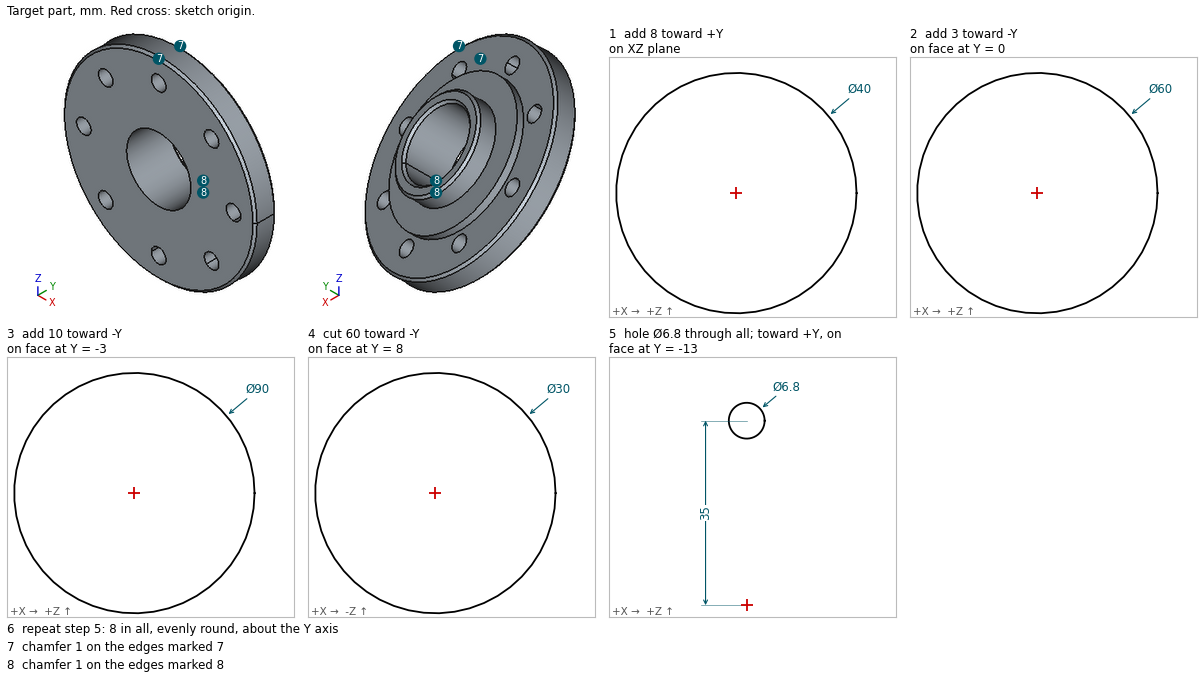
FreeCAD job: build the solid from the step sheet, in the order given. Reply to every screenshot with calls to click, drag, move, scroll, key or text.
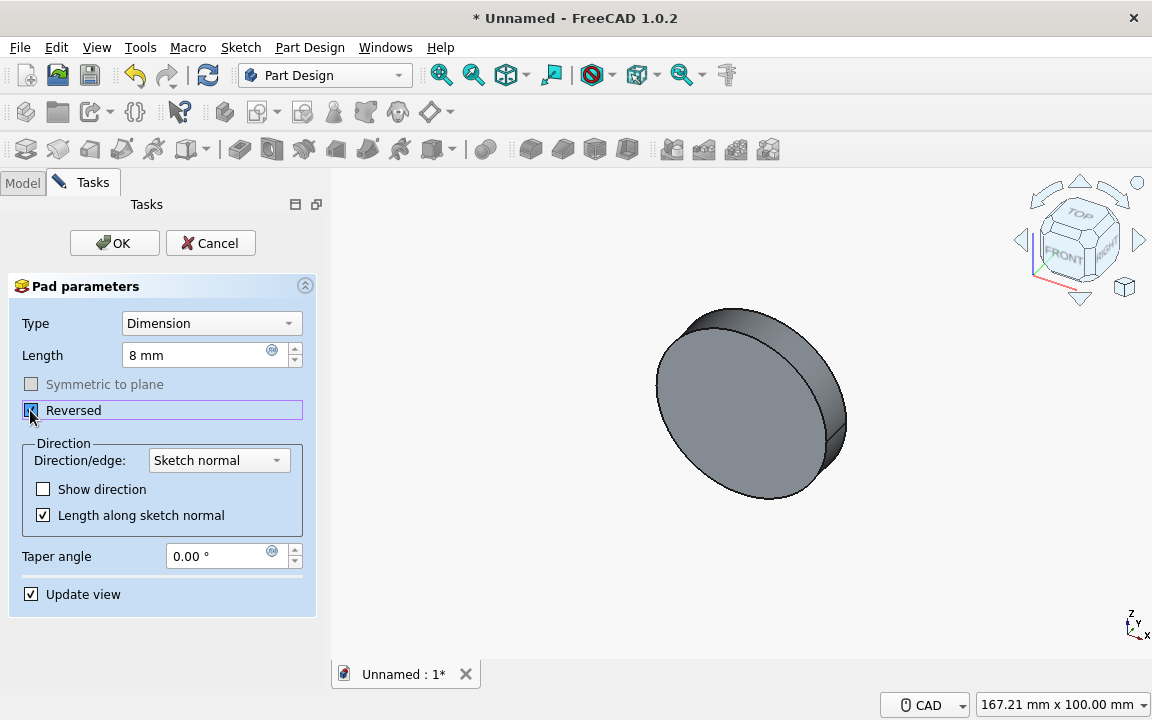
click(115, 243)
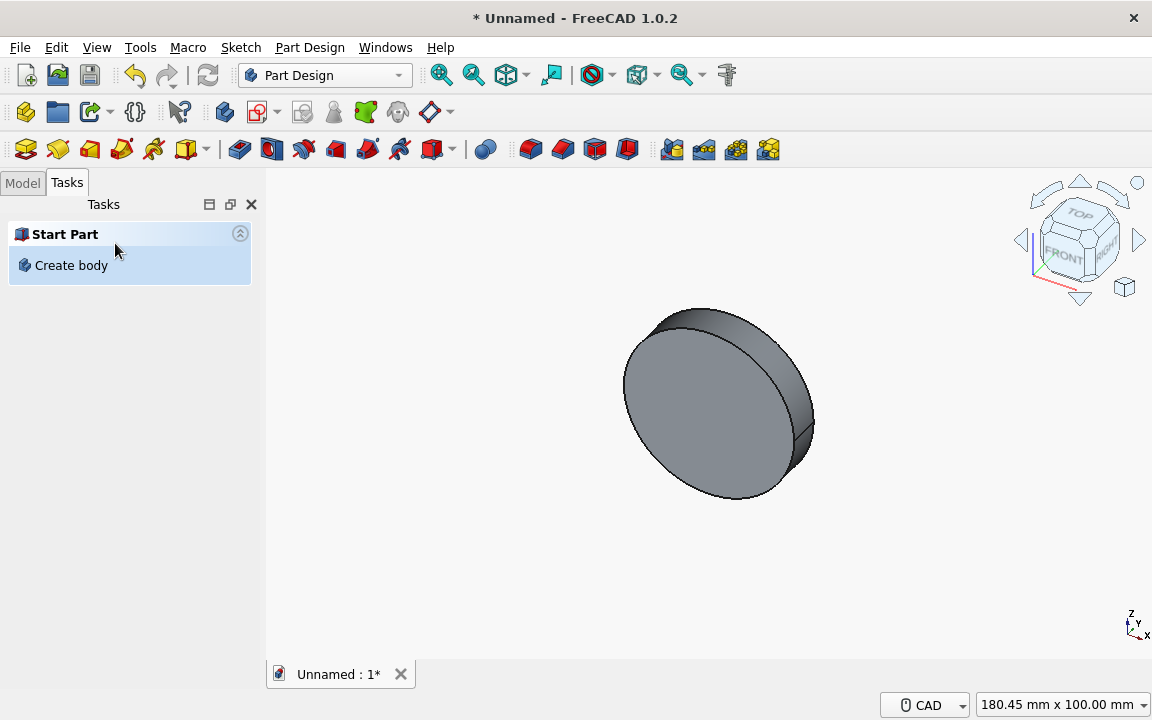
click(709, 412)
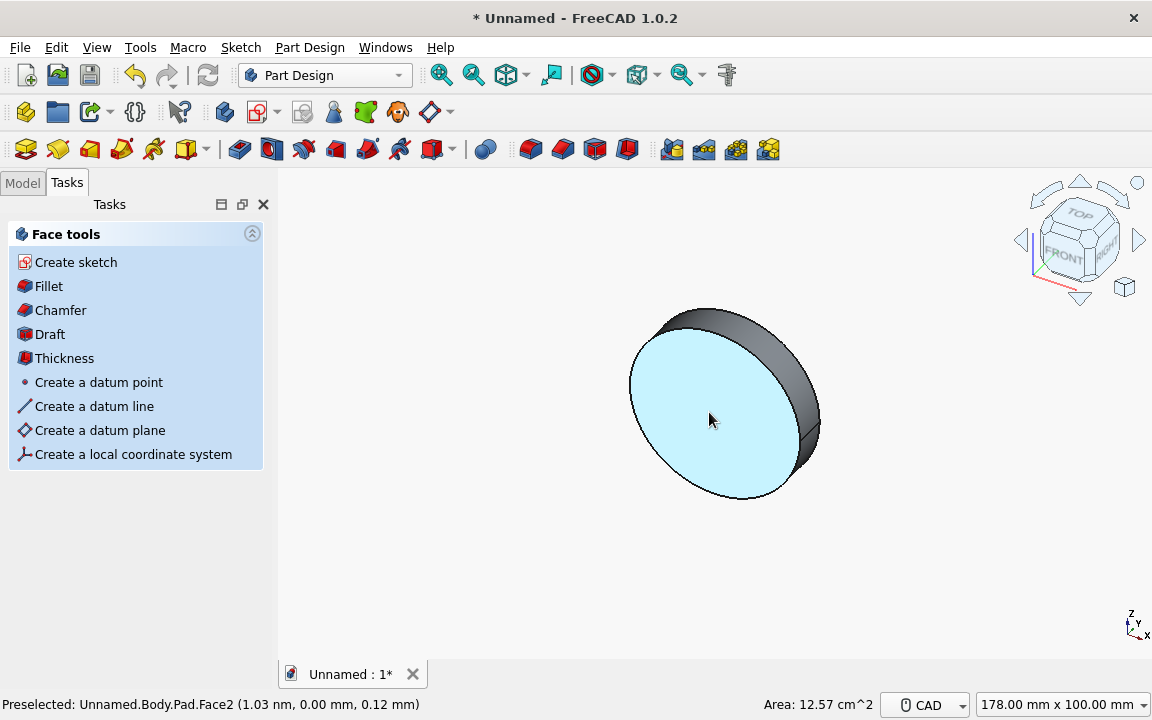
click(258, 112)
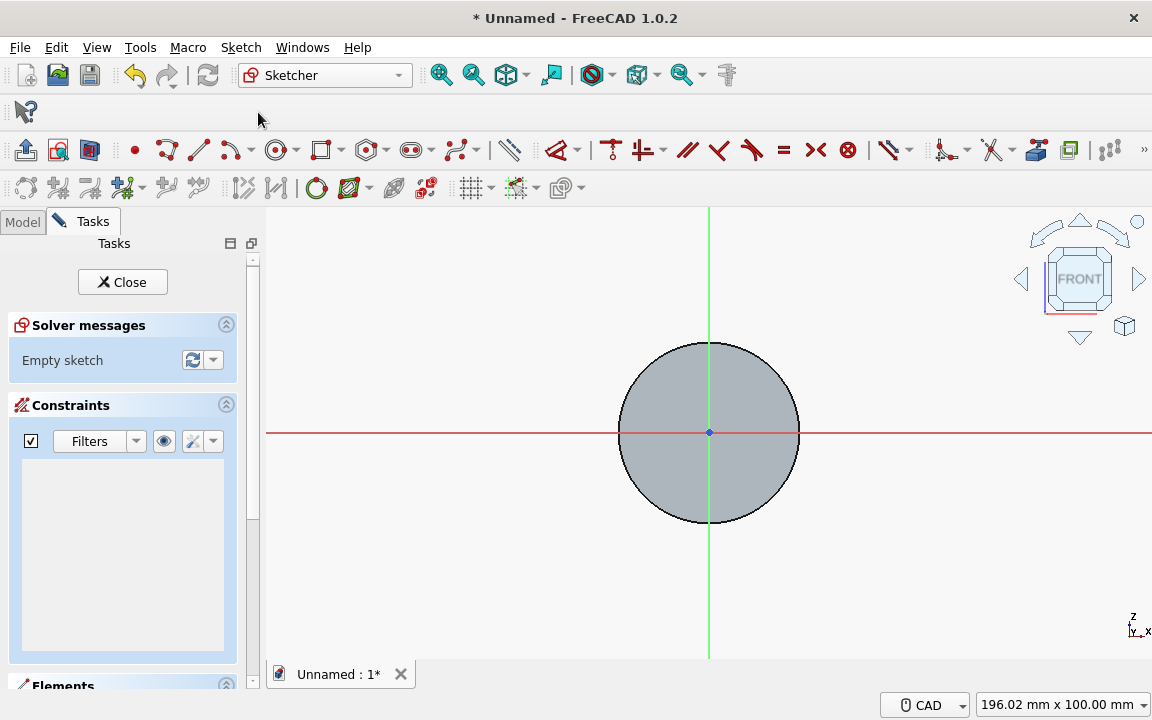
click(276, 150)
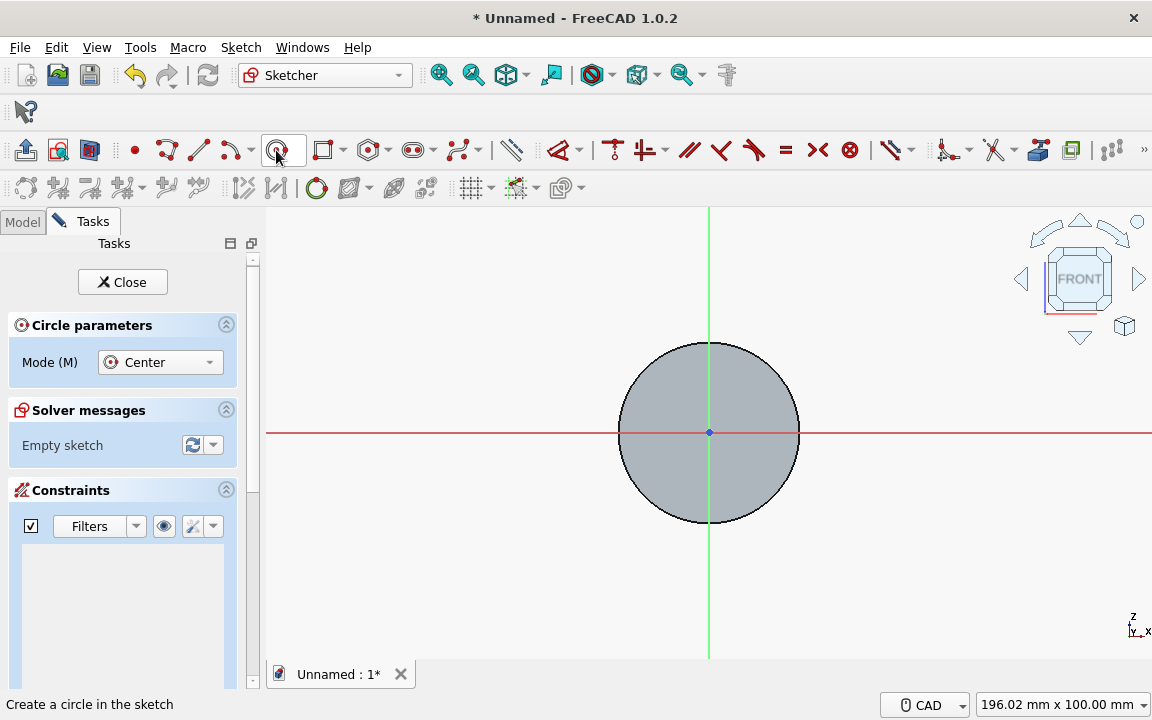
click(709, 433)
move(805, 337)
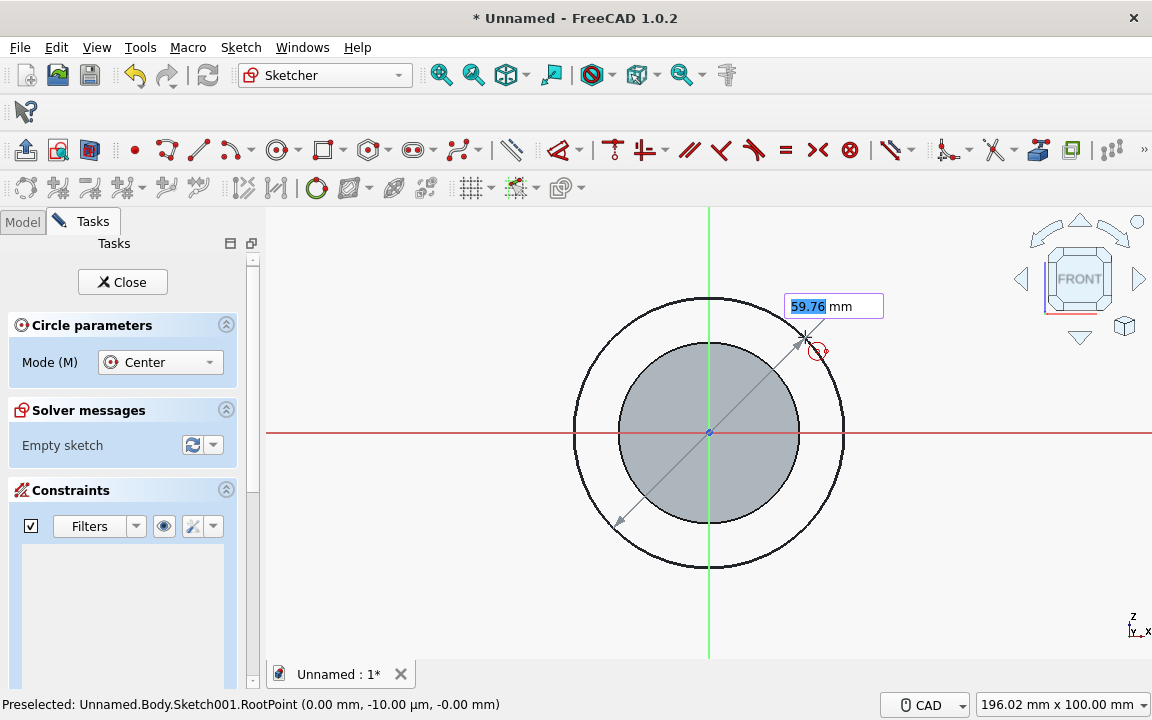
text(60)
key(Return)
key(Escape)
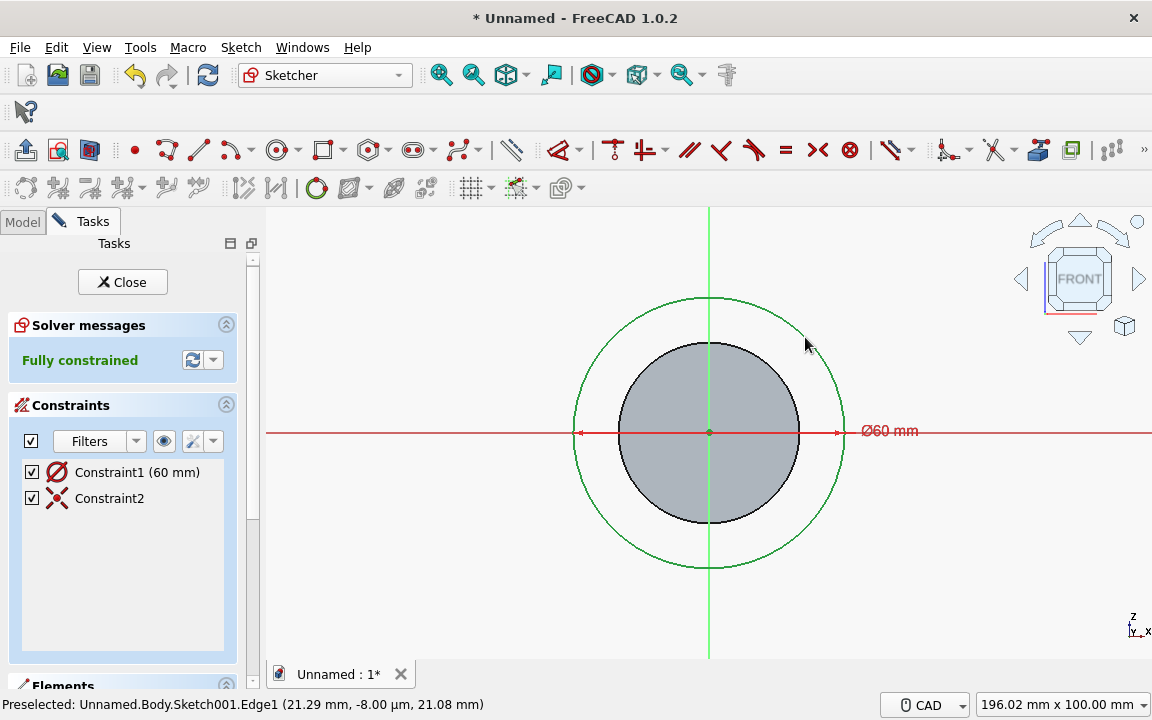
click(123, 282)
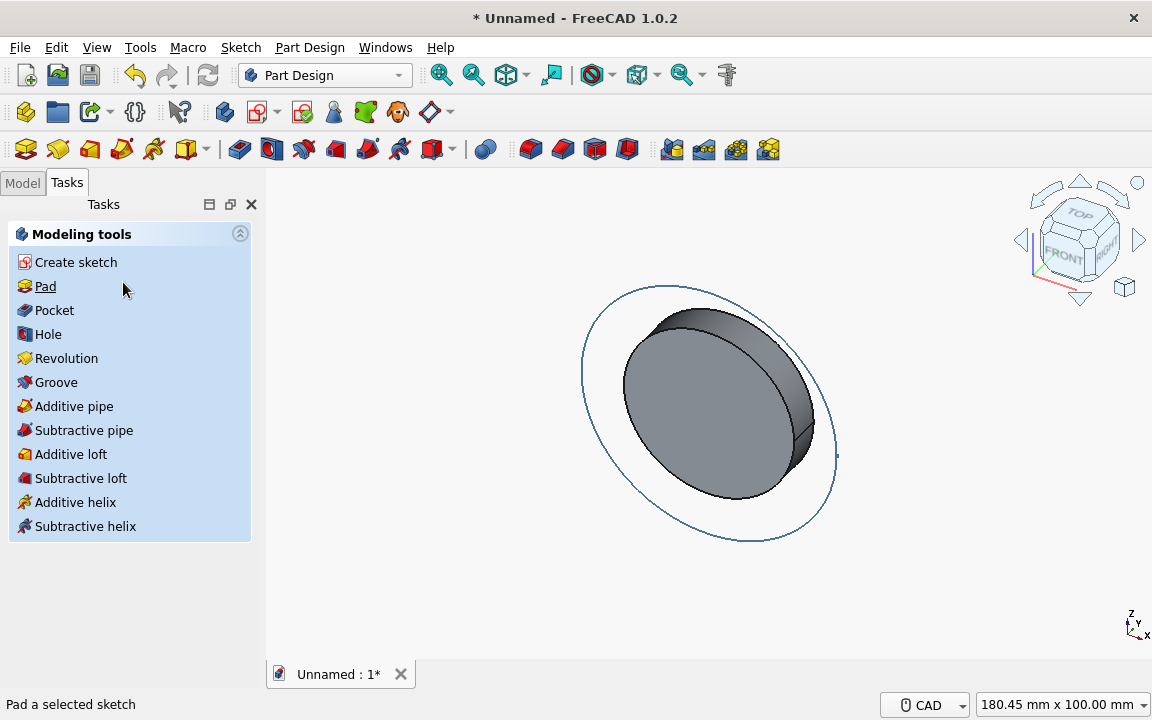
click(26, 150)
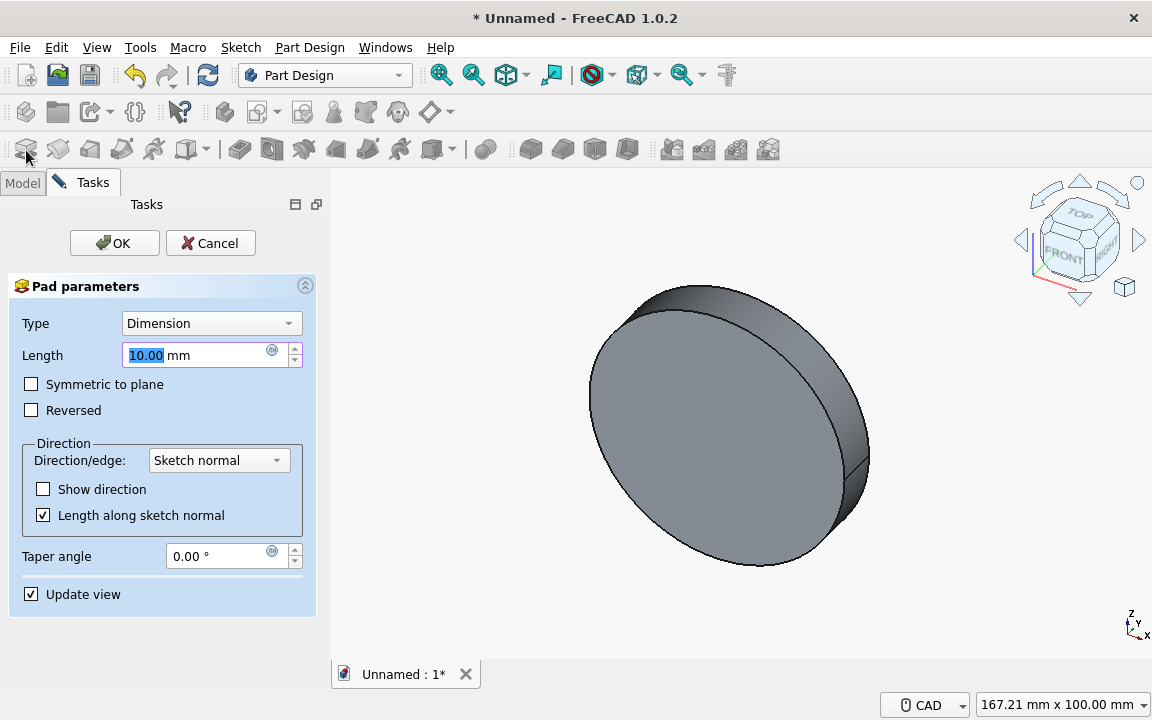
text(3)
key(Tab)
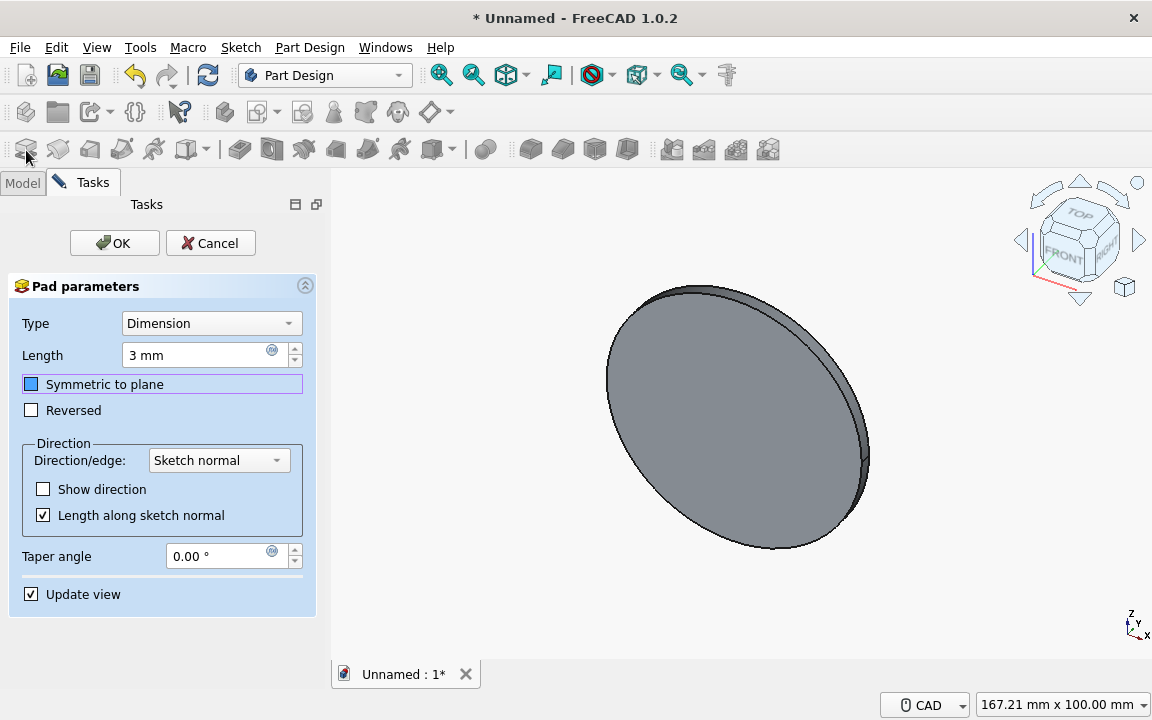
click(115, 243)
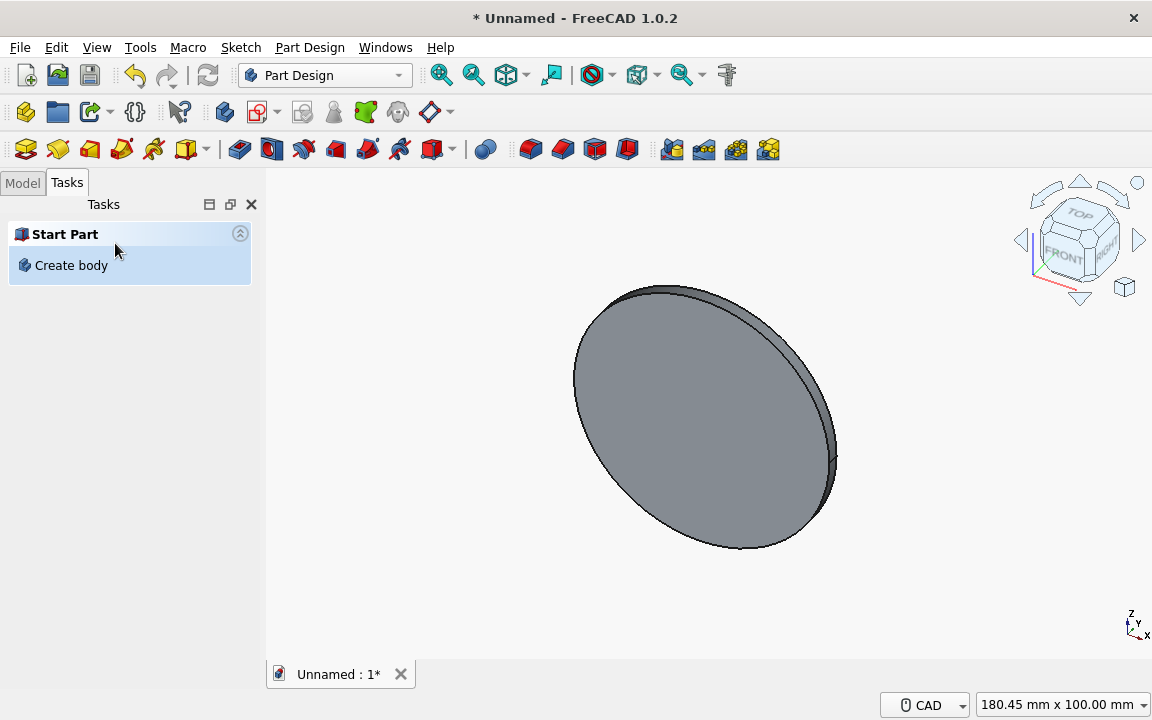
click(702, 420)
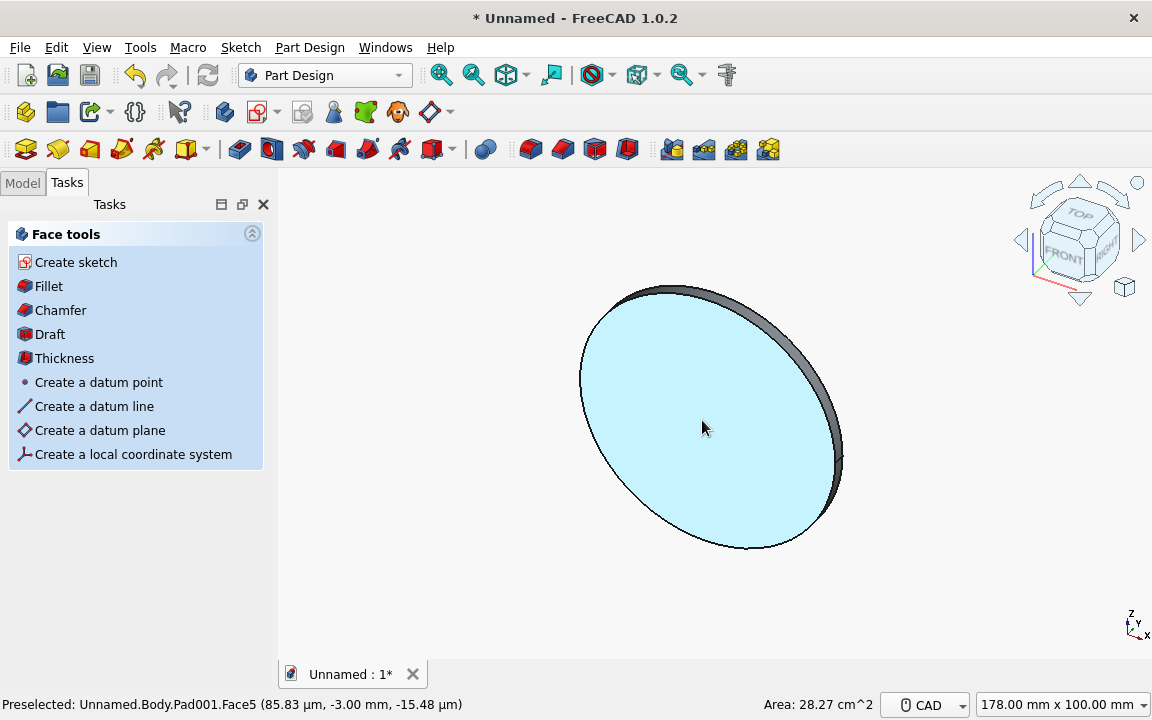
click(258, 112)